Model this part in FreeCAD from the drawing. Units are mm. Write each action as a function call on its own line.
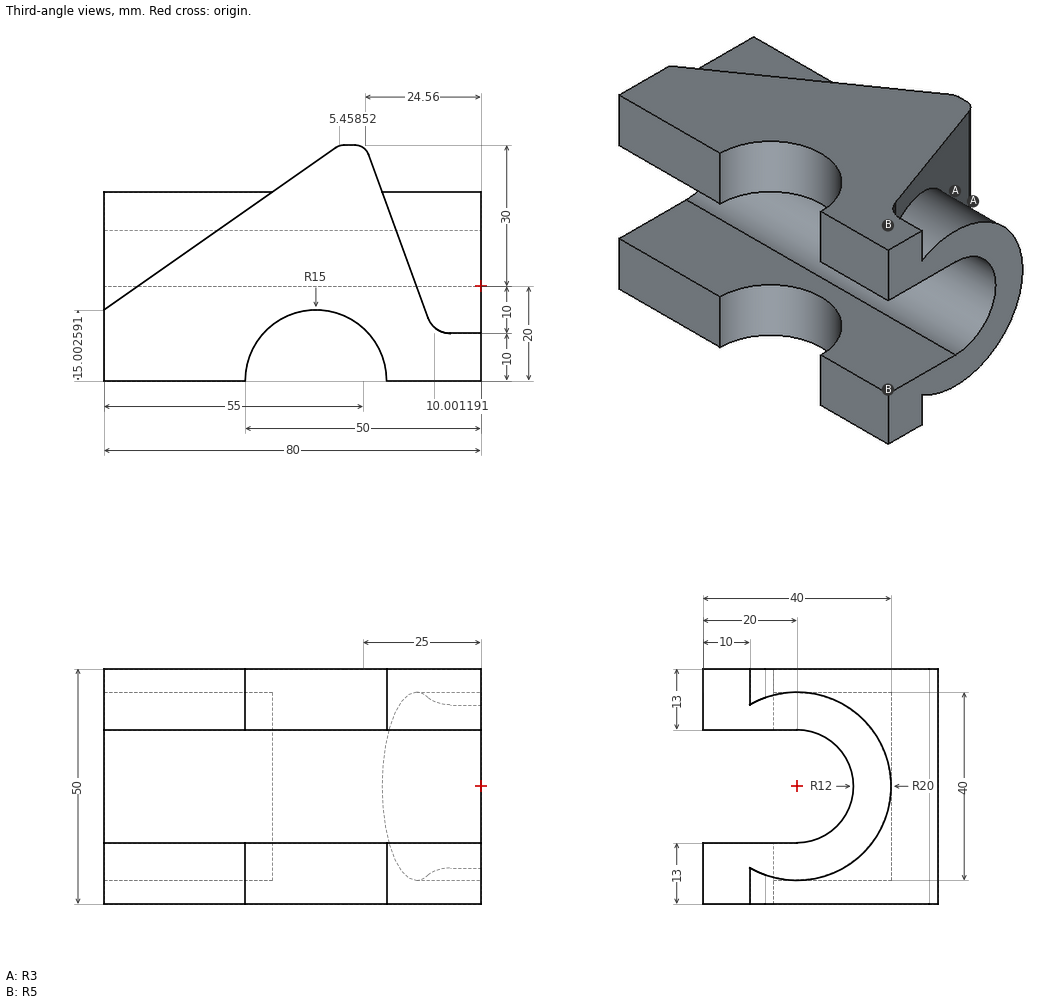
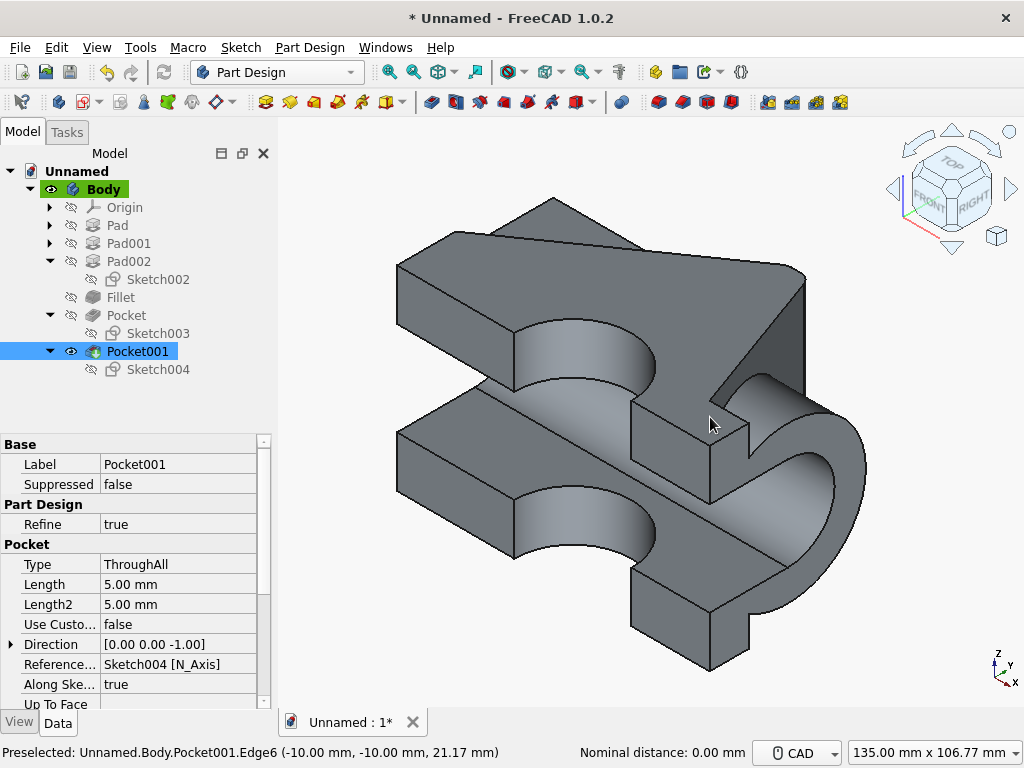
click(660, 102)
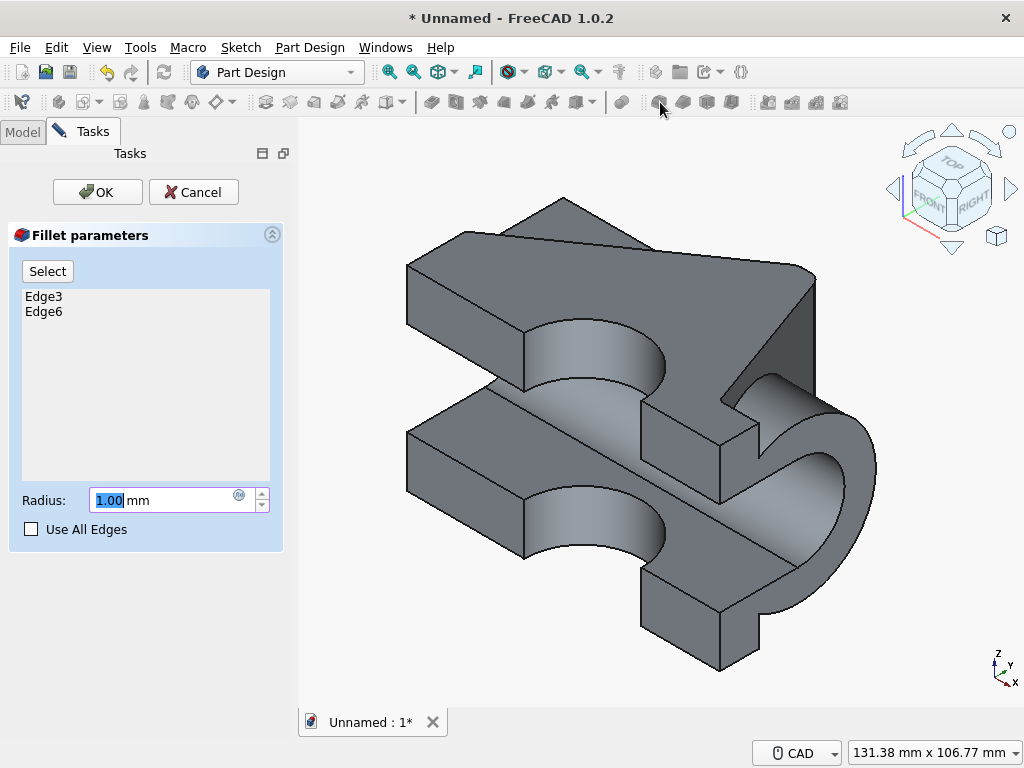
text(5)
key(Tab)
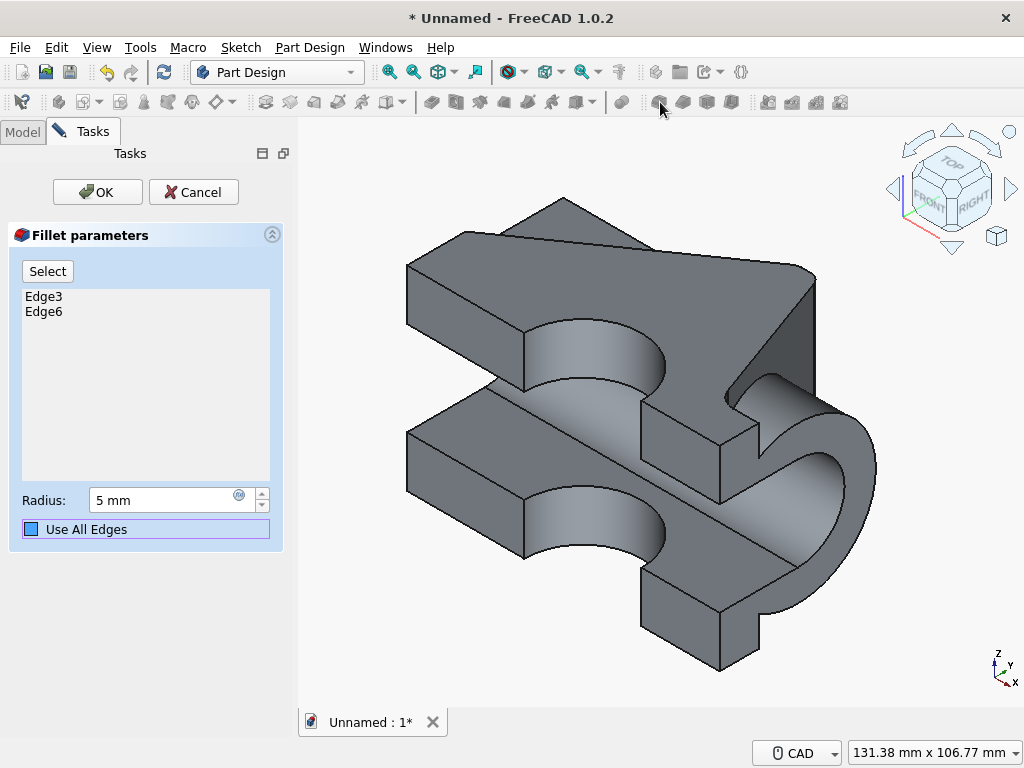
click(98, 192)